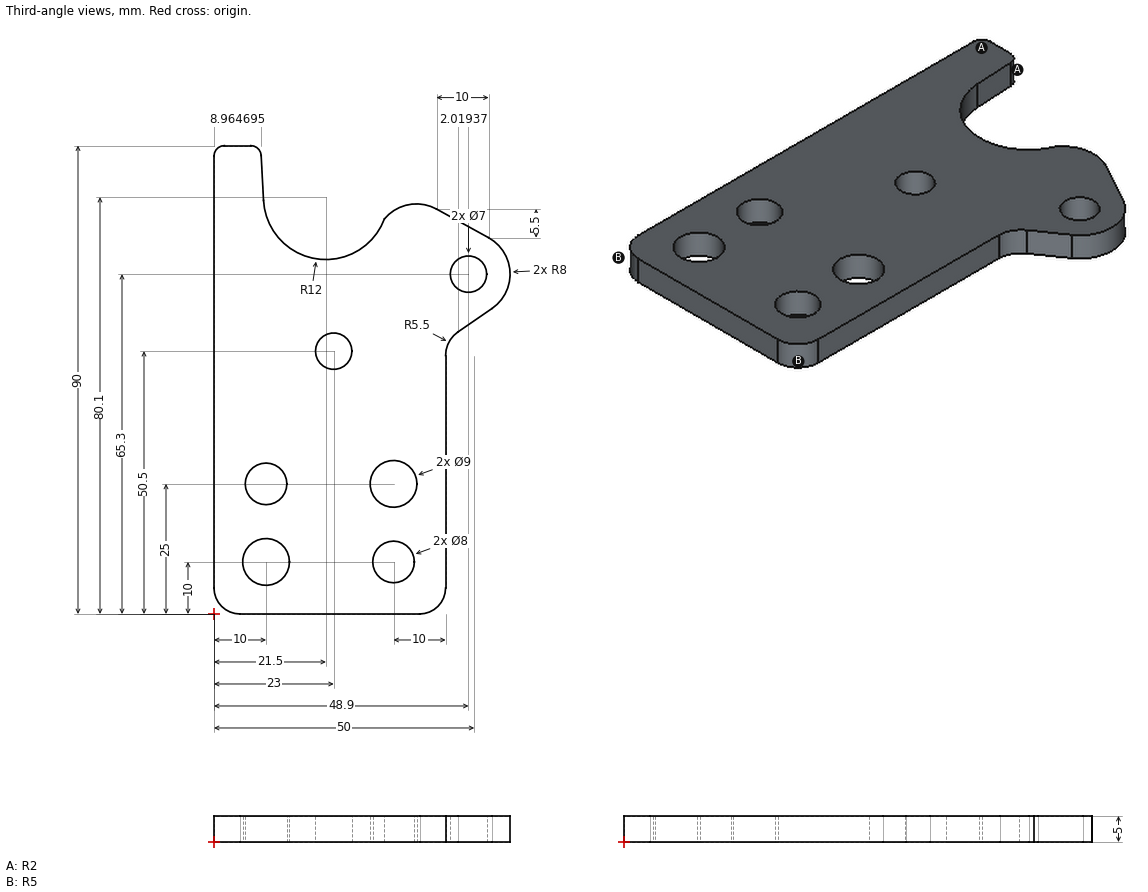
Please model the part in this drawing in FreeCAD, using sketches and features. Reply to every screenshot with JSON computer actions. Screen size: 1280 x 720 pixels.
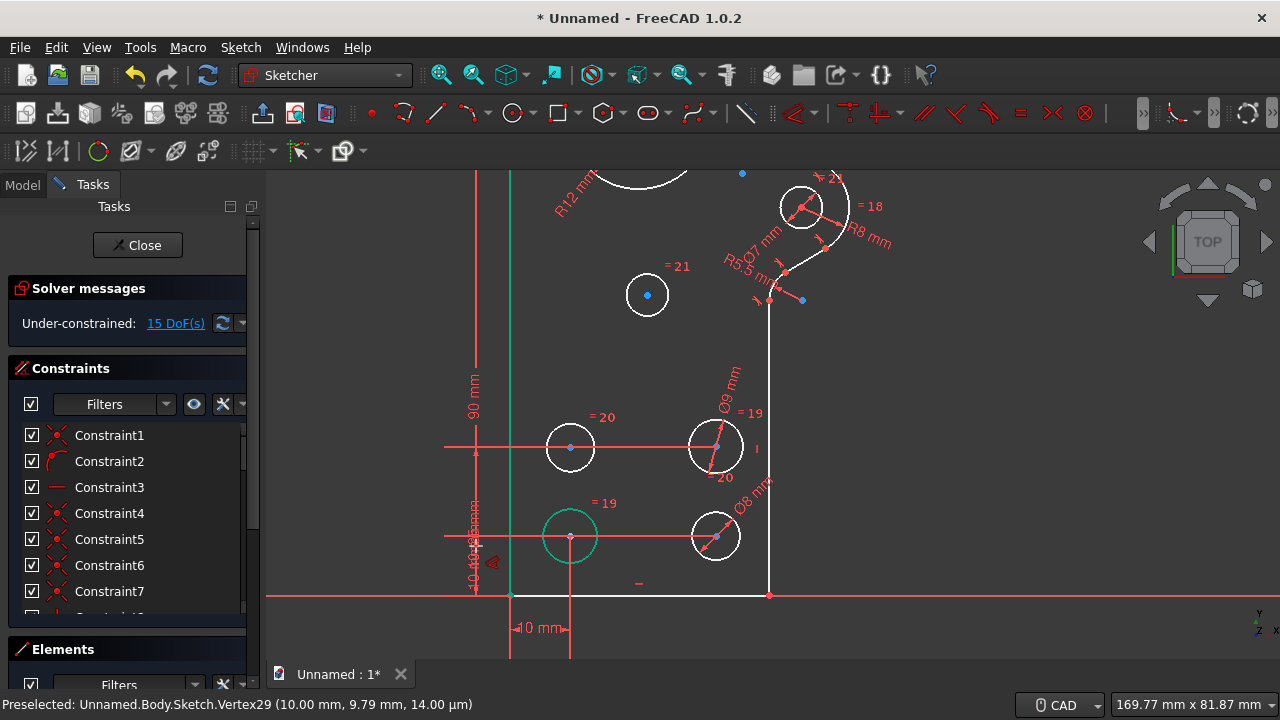
{"action": "left_click", "coordinate": [571, 448]}
{"action": "left_click", "coordinate": [554, 414]}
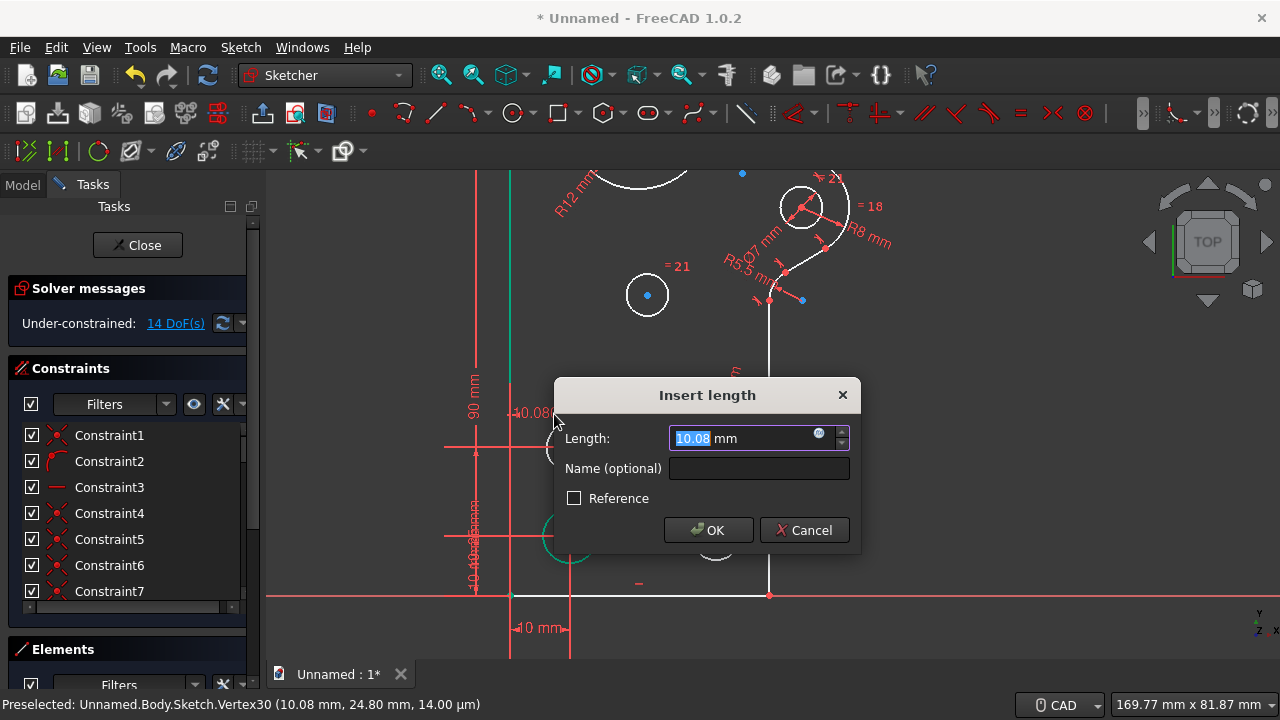
{"action": "type", "text": "10"}
{"action": "key", "text": "Return"}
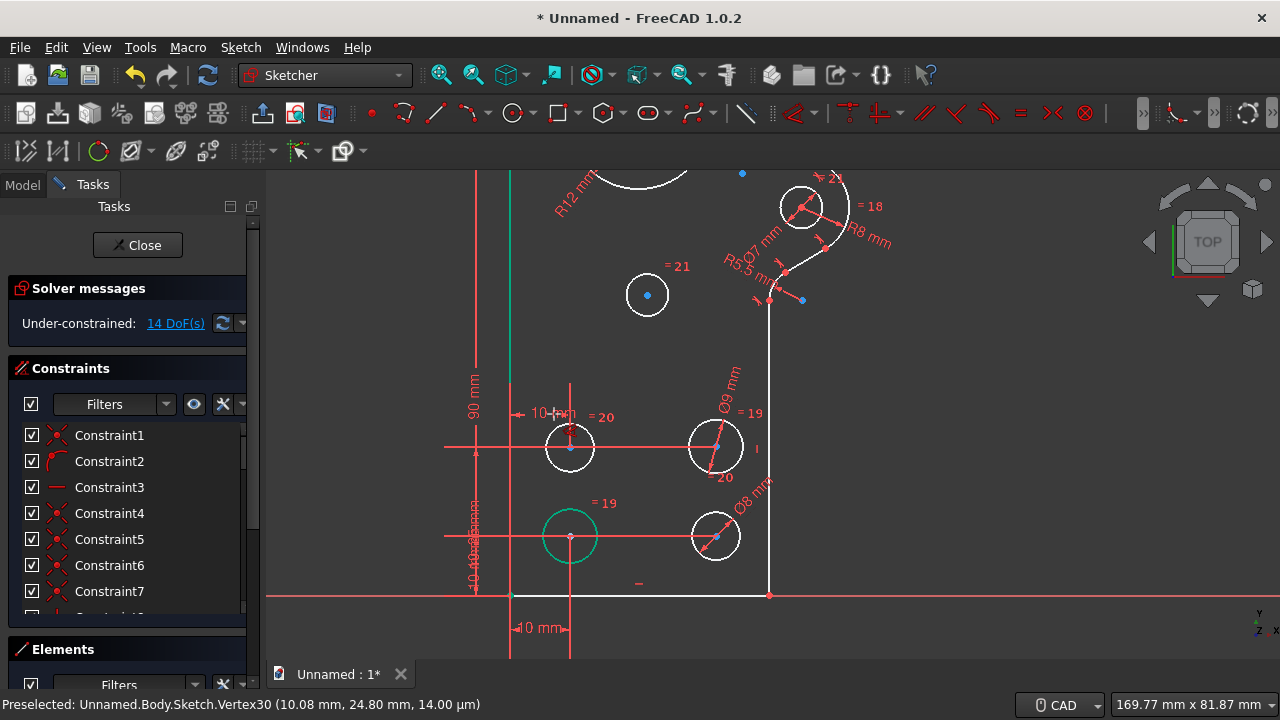
{"action": "left_click", "coordinate": [570, 448]}
{"action": "left_click", "coordinate": [476, 488]}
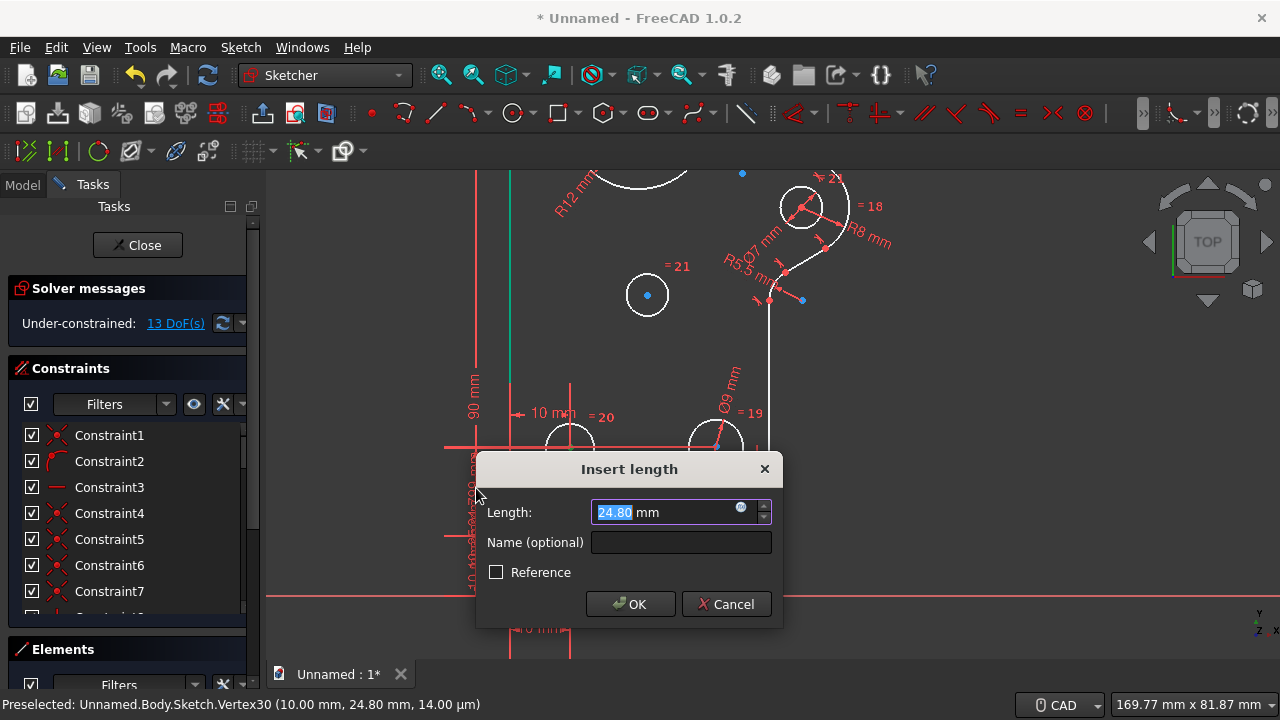
{"action": "type", "text": "25"}
{"action": "key", "text": "Return"}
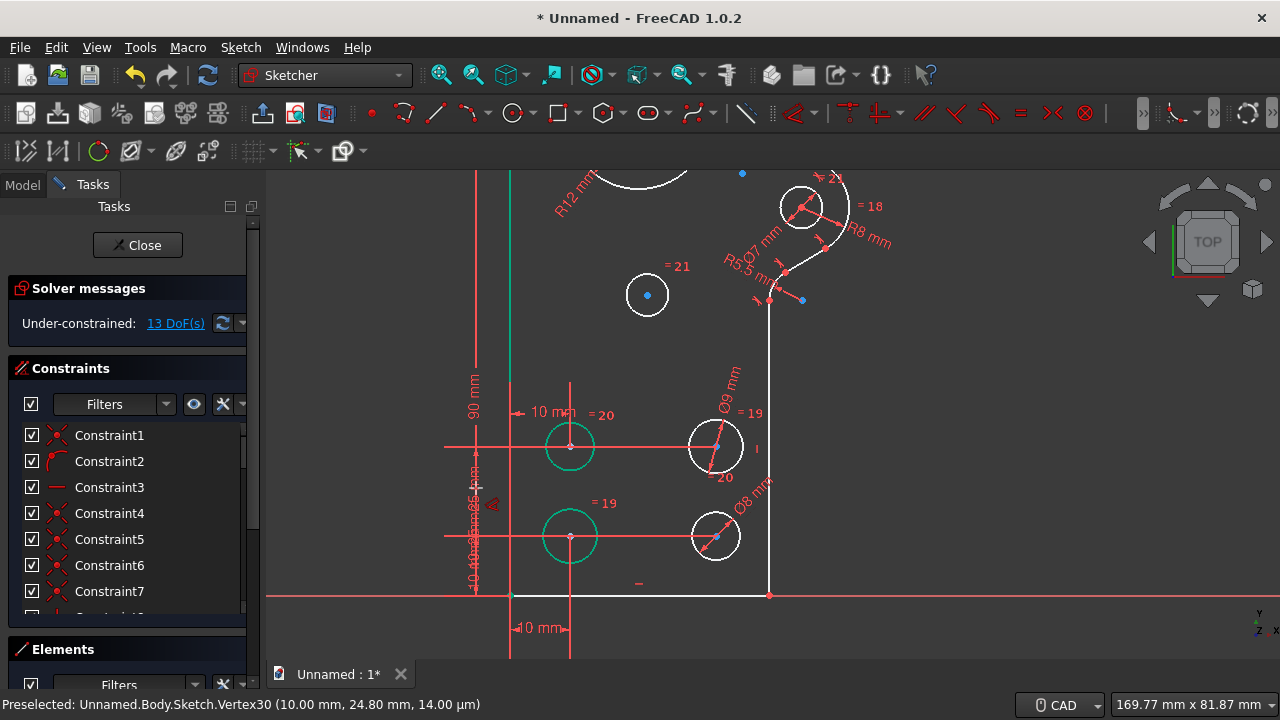
{"action": "left_click", "coordinate": [647, 295]}
{"action": "left_click", "coordinate": [627, 630]}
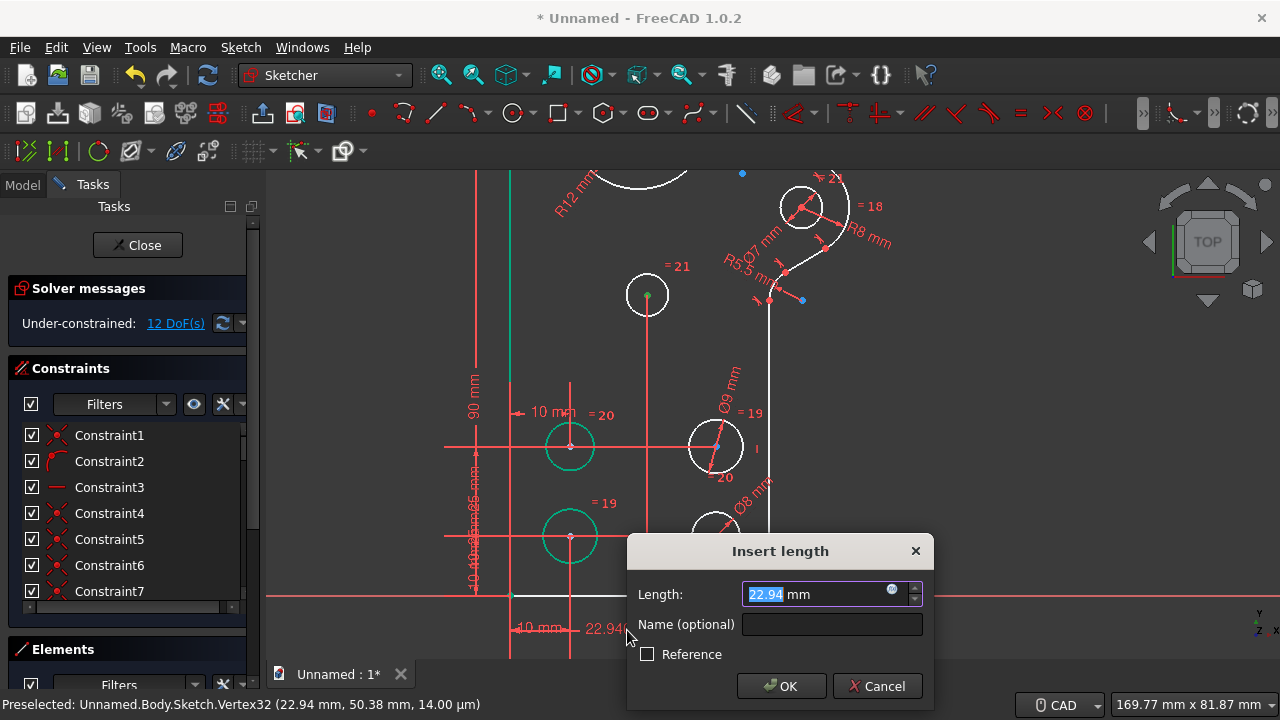
{"action": "type", "text": "23"}
{"action": "key", "text": "Return"}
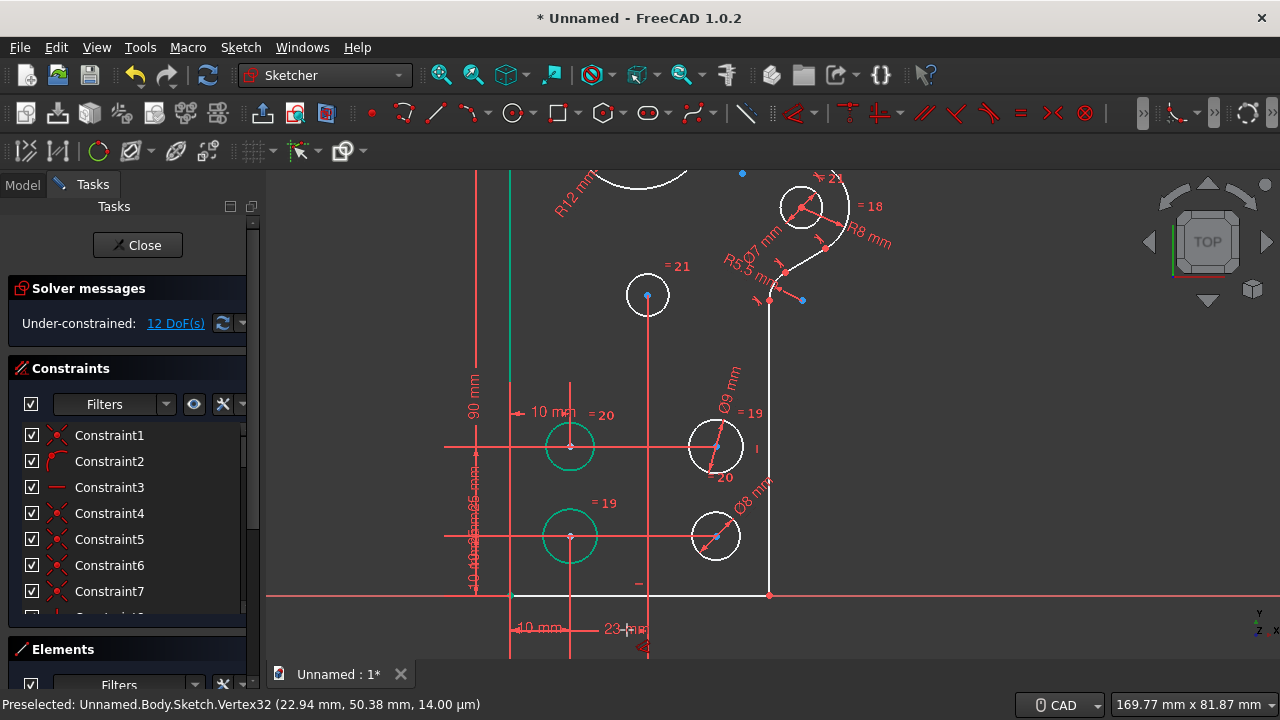
{"action": "scroll", "coordinate": [734, 521], "scroll_direction": "down", "scroll_amount": 3}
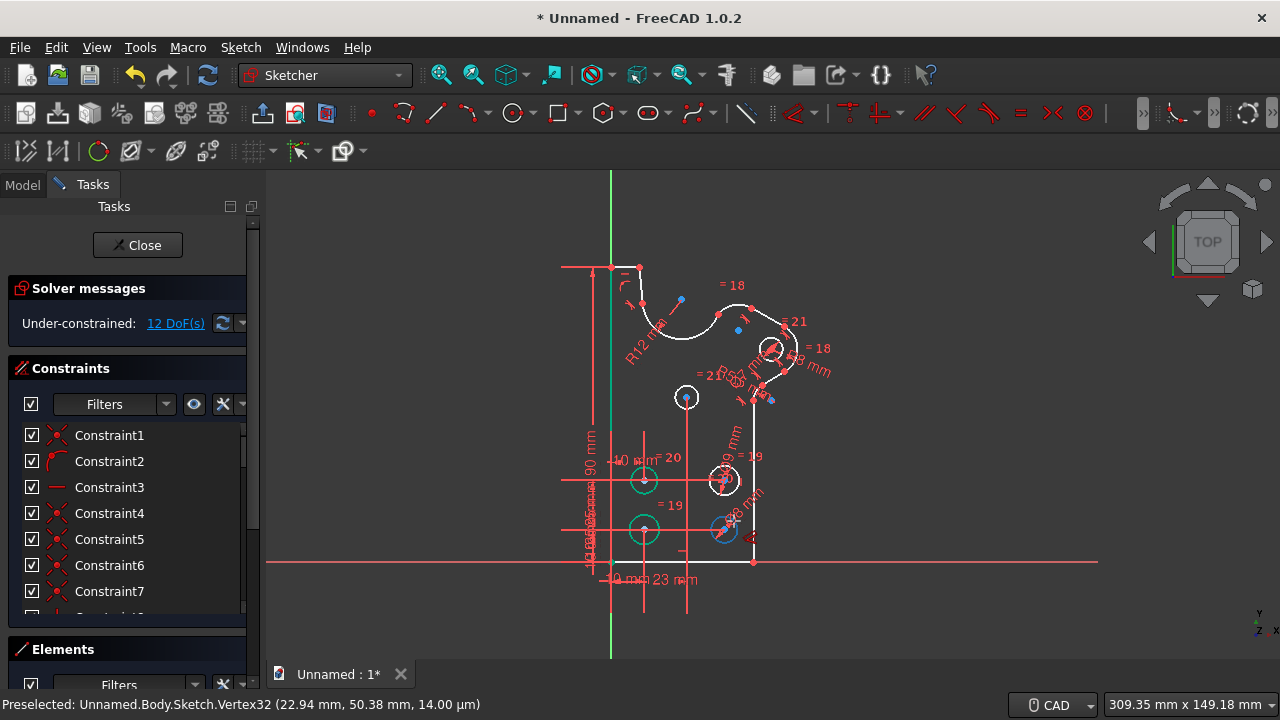
{"action": "scroll", "coordinate": [774, 321], "scroll_direction": "up", "scroll_amount": 2}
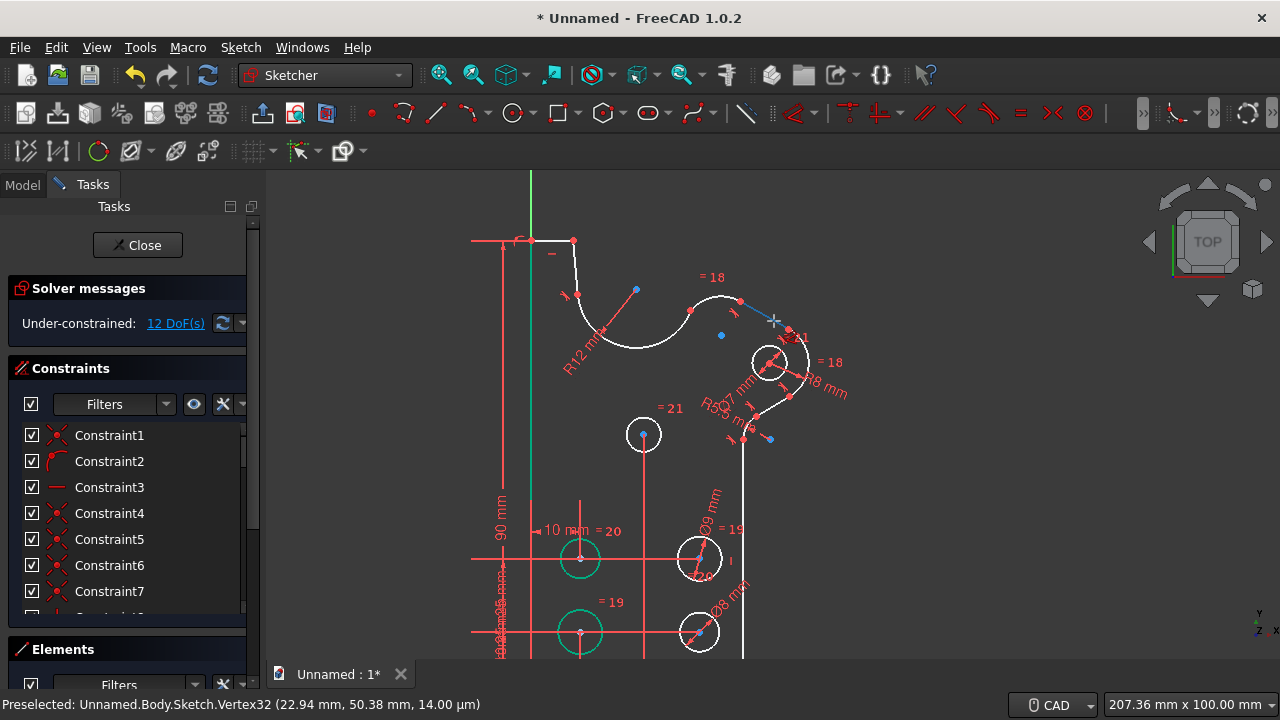
{"action": "left_click", "coordinate": [774, 321]}
{"action": "left_click", "coordinate": [765, 268]}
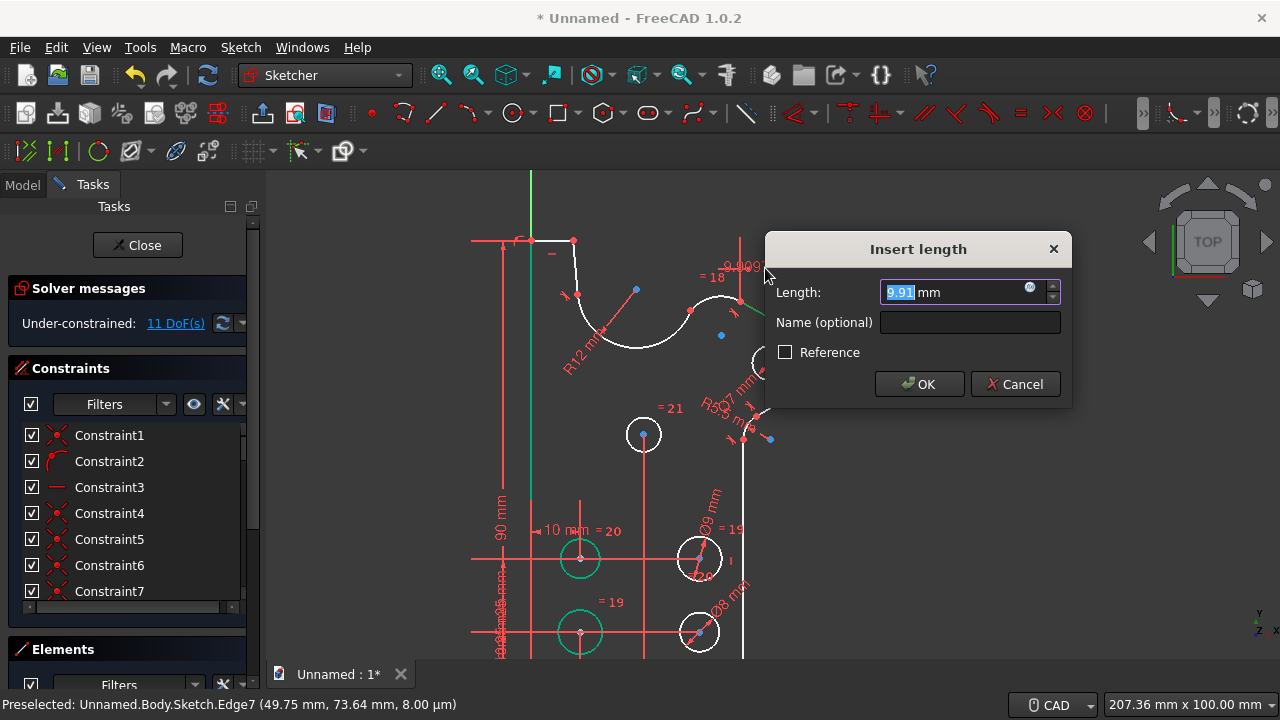
{"action": "type", "text": "10"}
{"action": "key", "text": "Return"}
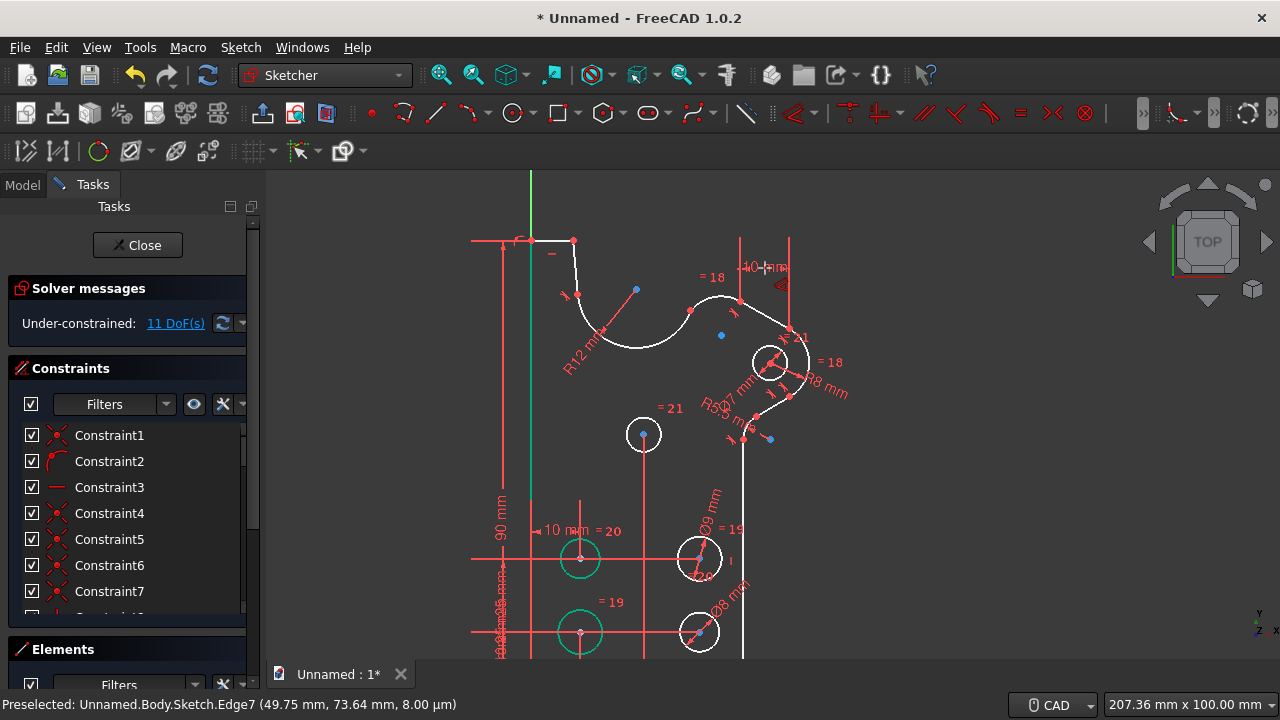
{"action": "left_click", "coordinate": [770, 440]}
{"action": "left_click", "coordinate": [596, 406]}